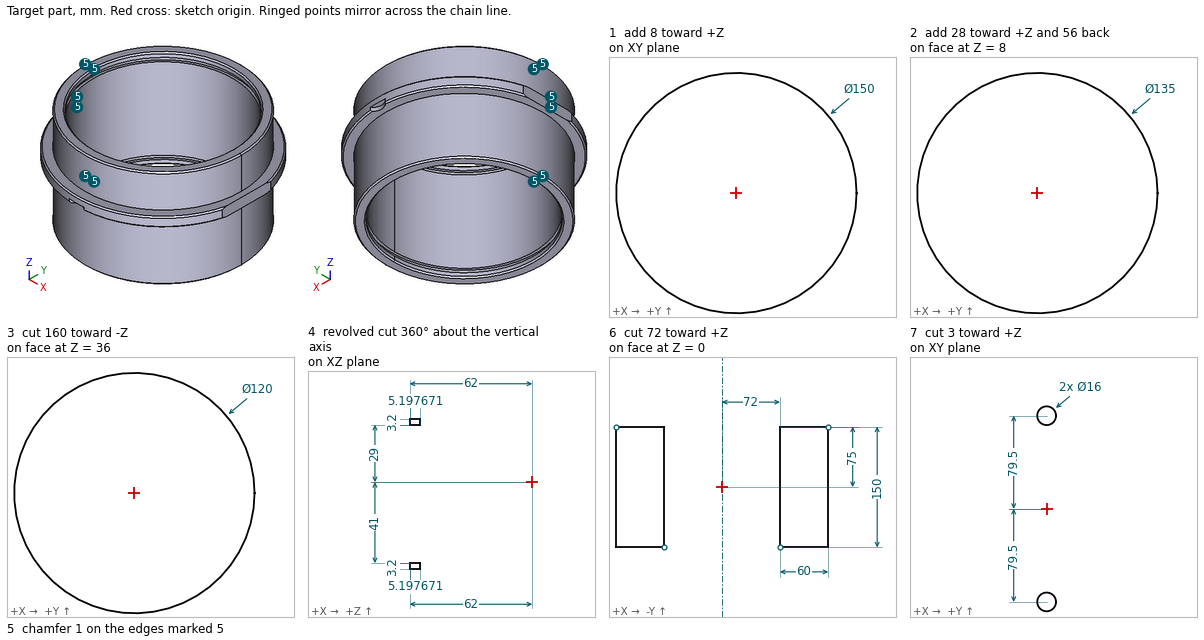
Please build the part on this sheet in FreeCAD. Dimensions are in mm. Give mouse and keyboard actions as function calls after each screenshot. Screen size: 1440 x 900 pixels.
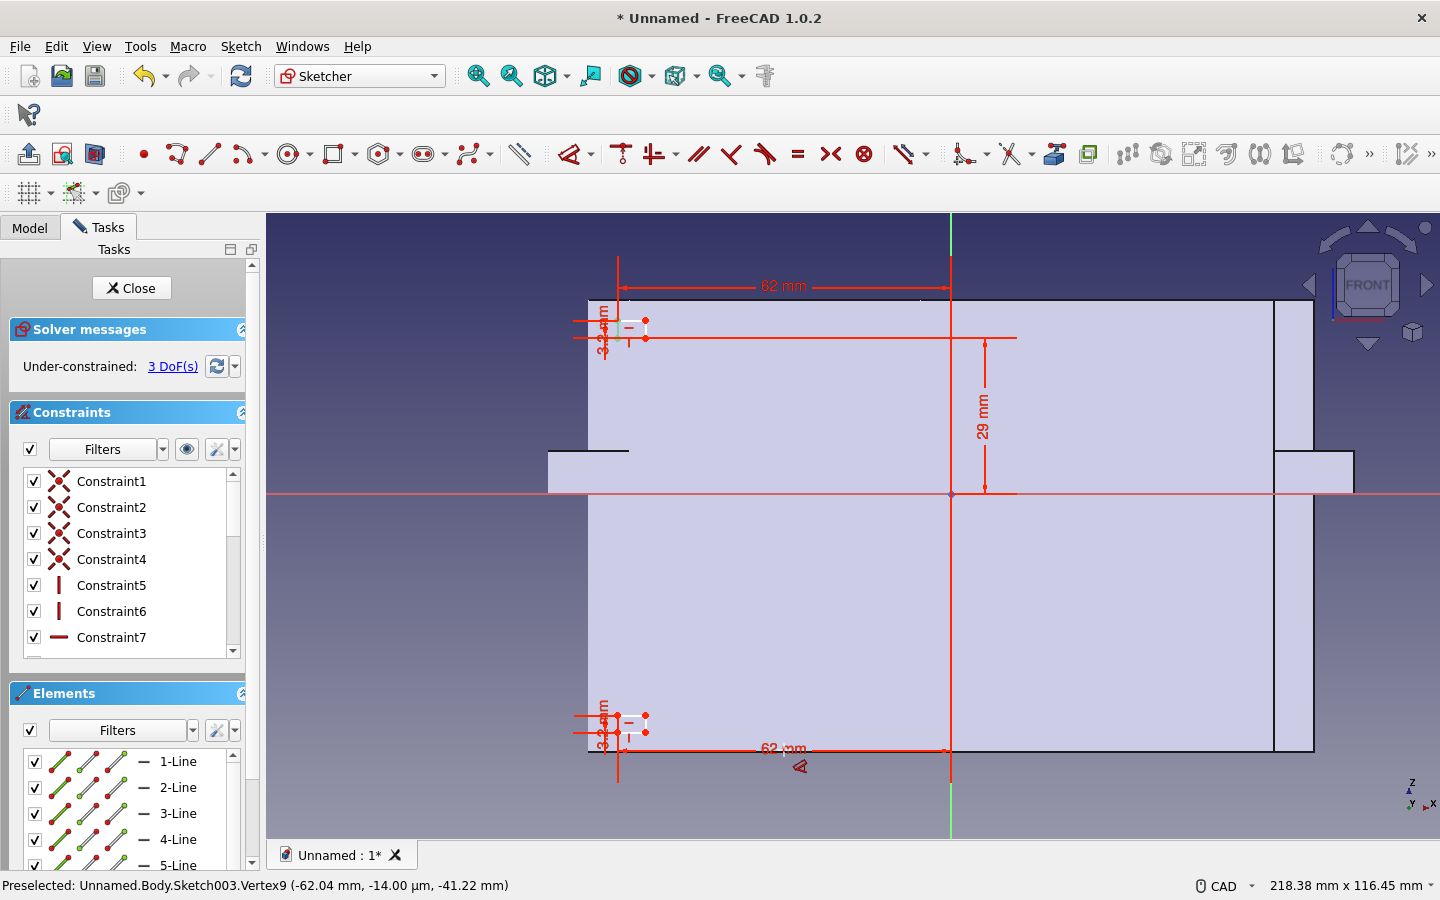
click(618, 716)
click(985, 605)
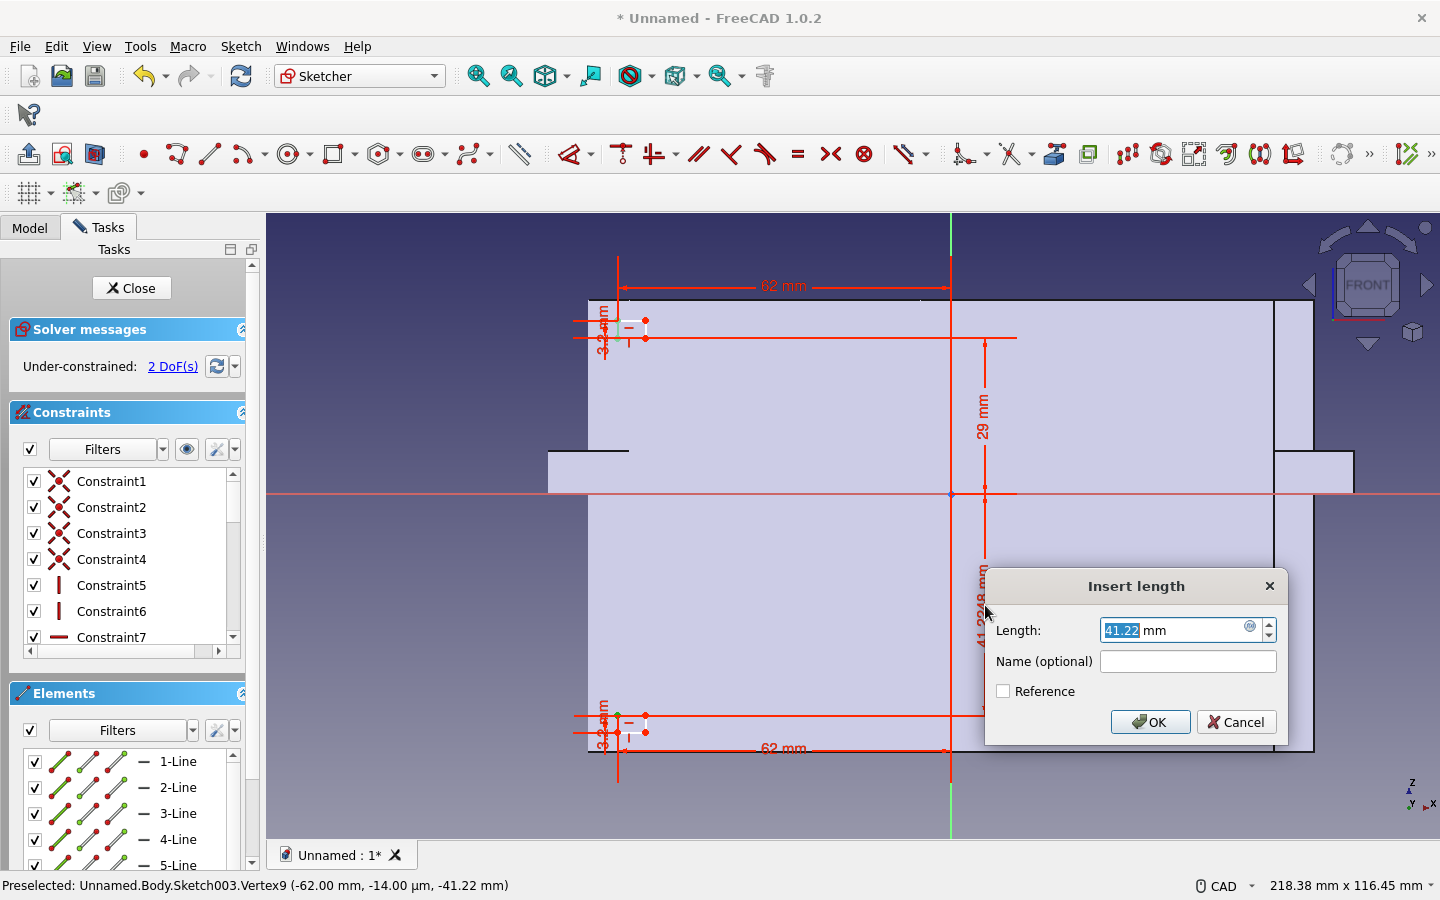
text(41)
key(Return)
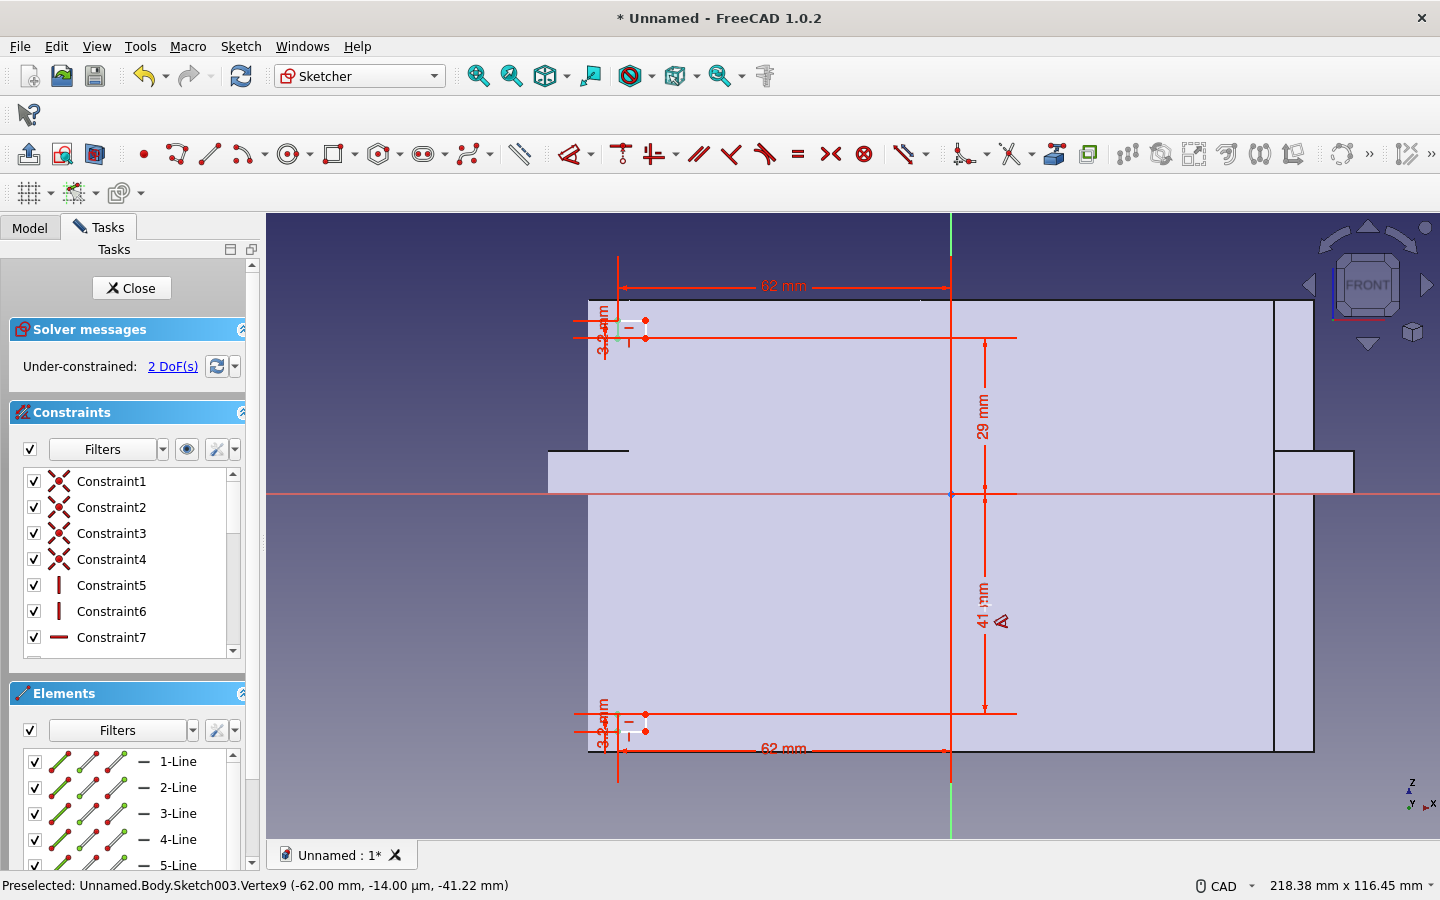
scroll(629, 338, up, 2)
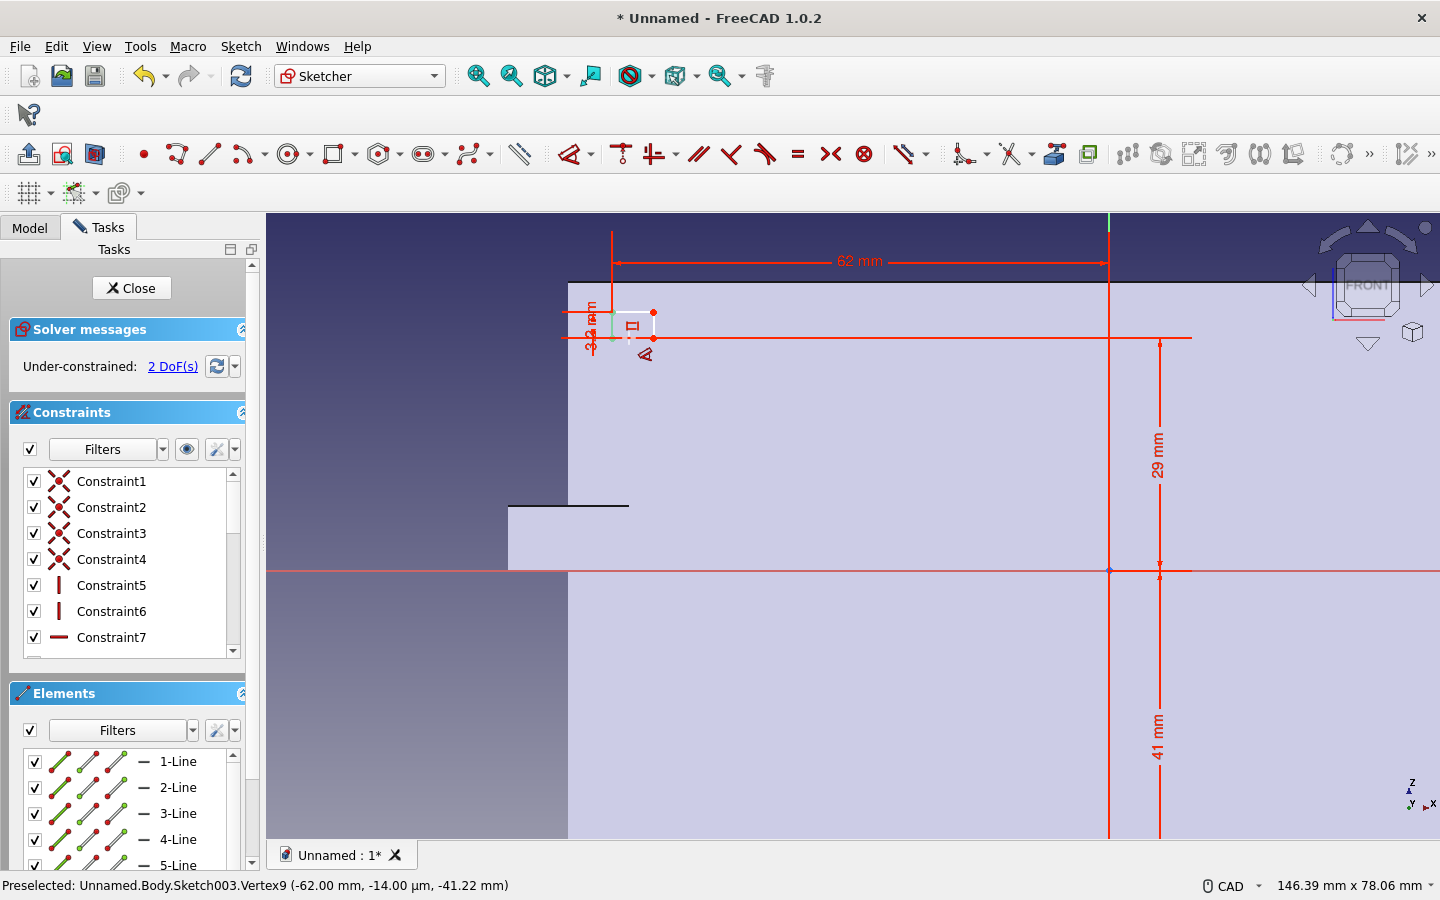
click(629, 338)
click(633, 372)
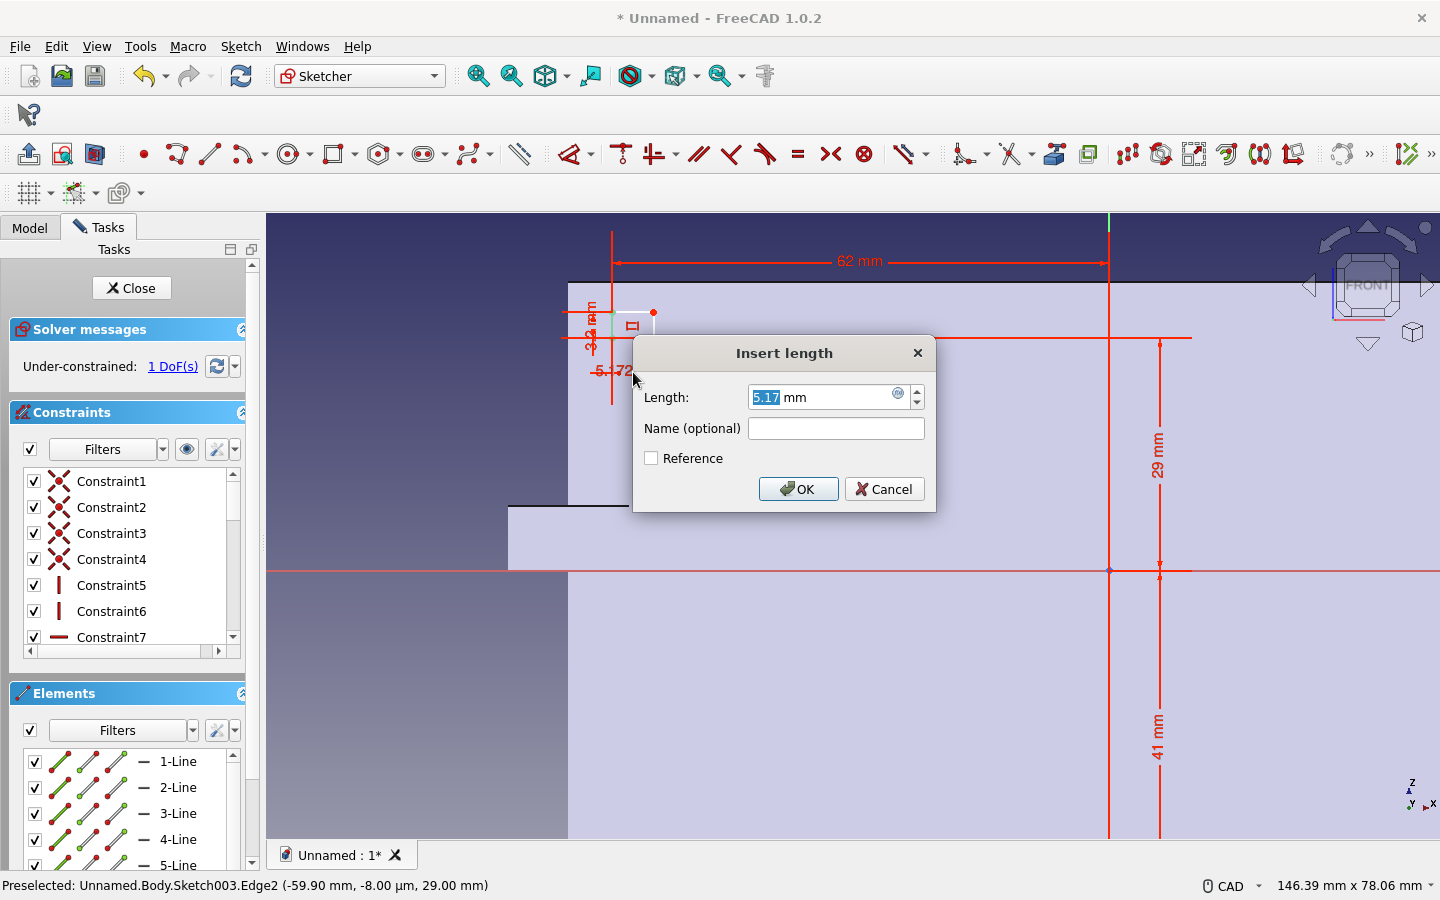
text(5.197671)
key(Return)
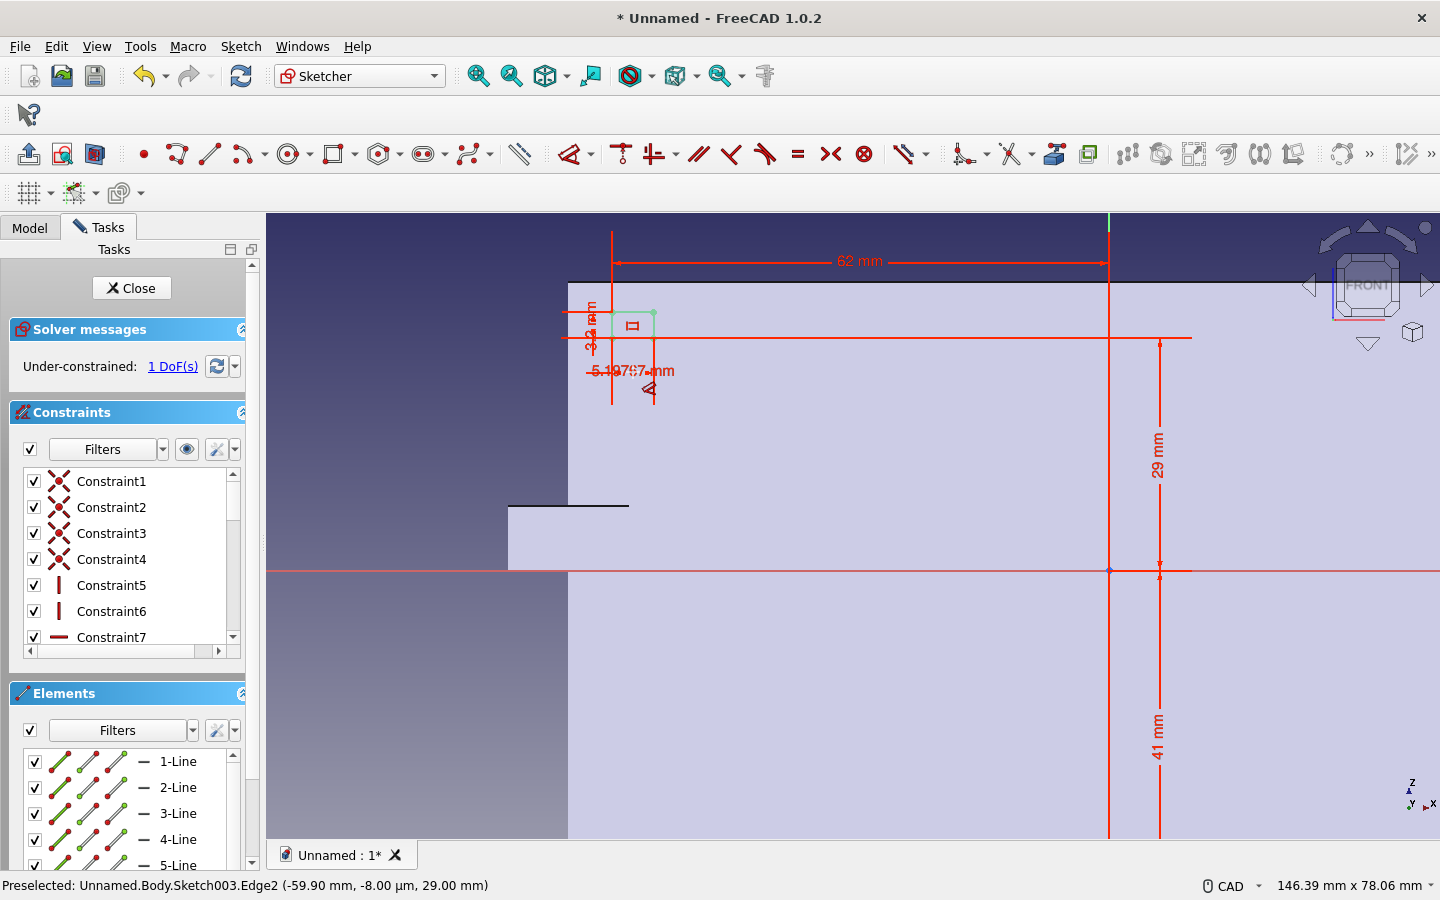
scroll(629, 337, down, 2)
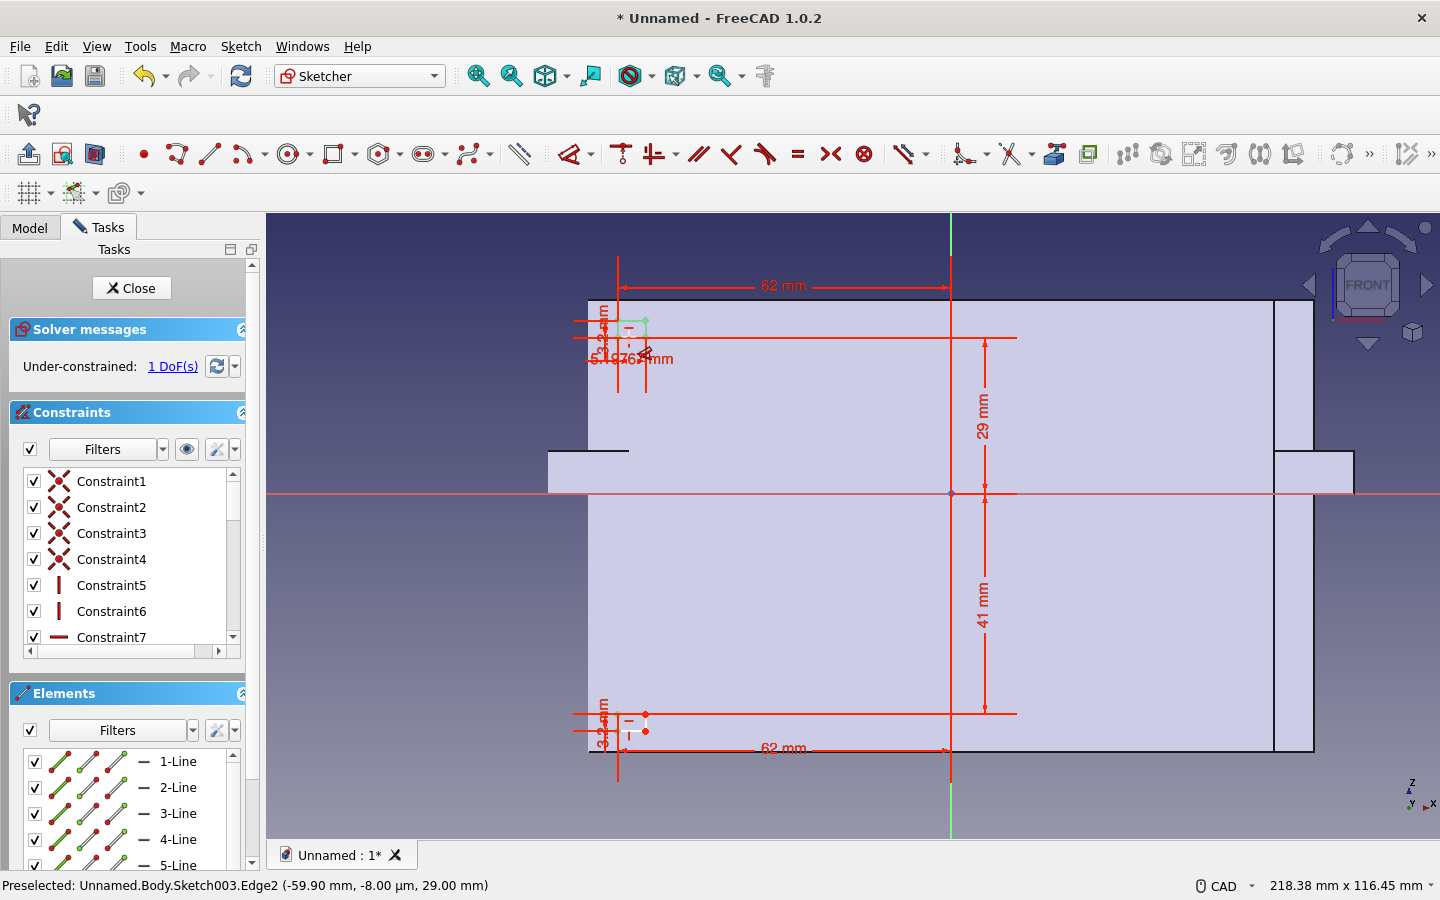
scroll(626, 731, up, 3)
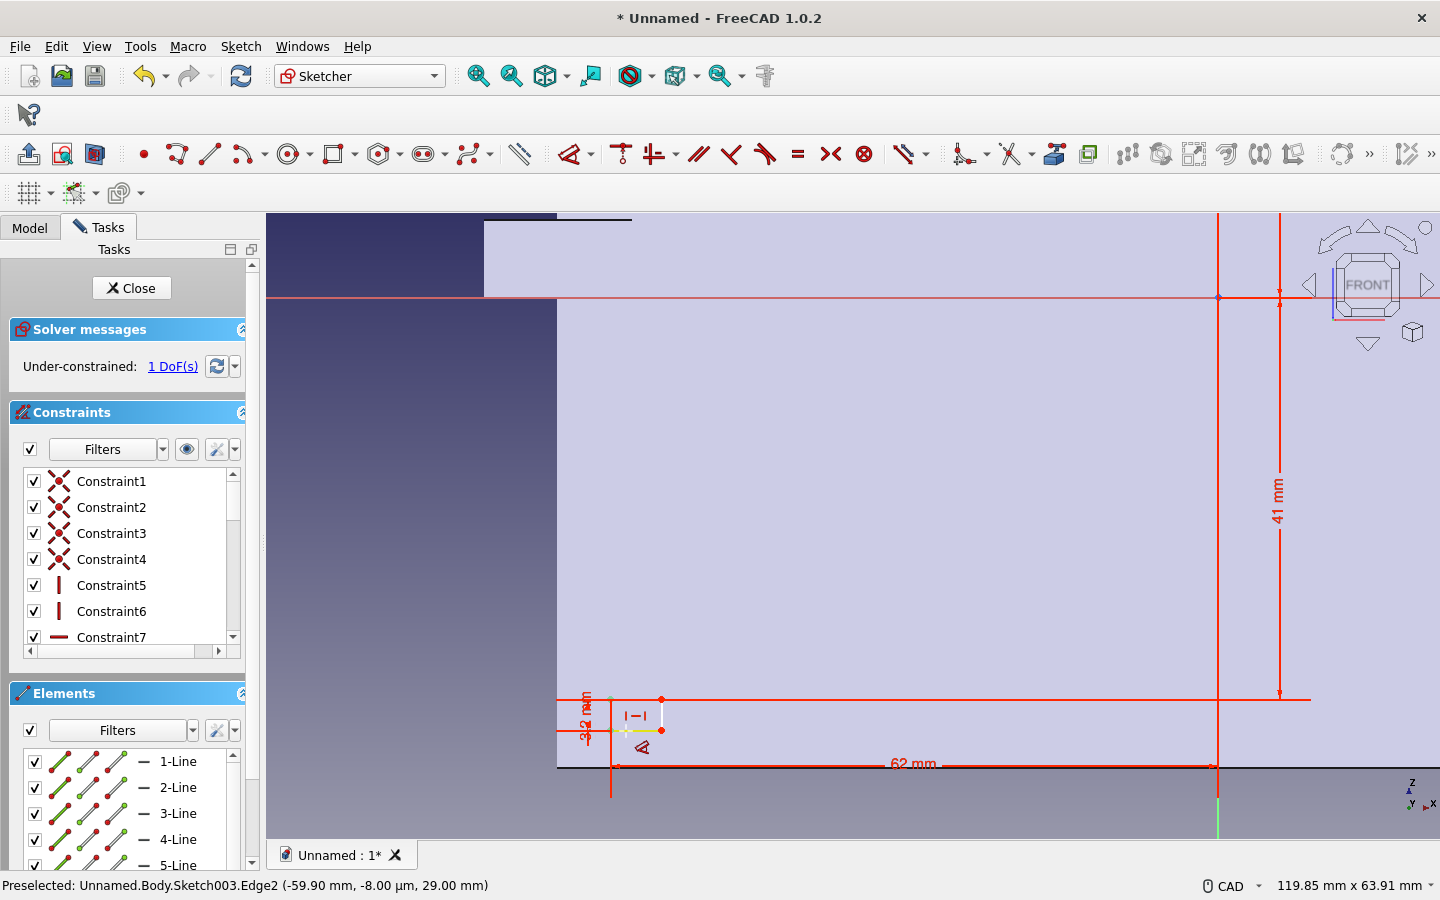
click(626, 731)
click(636, 765)